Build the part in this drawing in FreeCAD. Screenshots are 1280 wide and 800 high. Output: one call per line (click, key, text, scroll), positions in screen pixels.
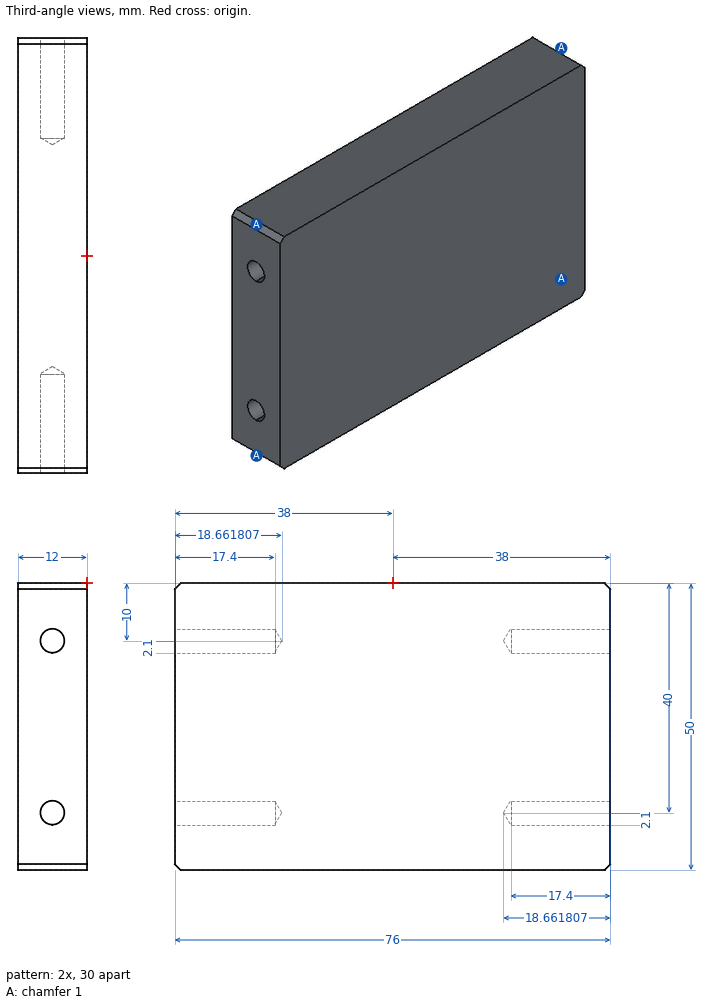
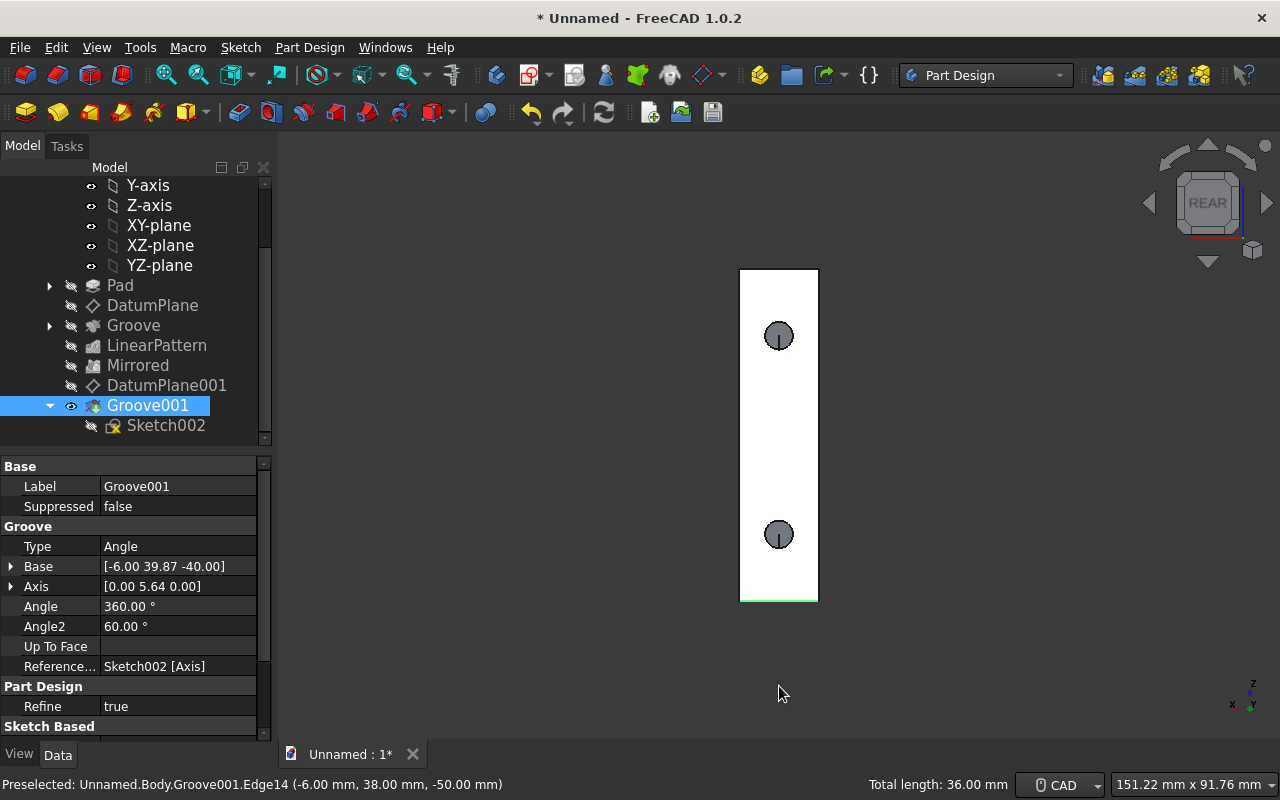
click(779, 268, ctrl)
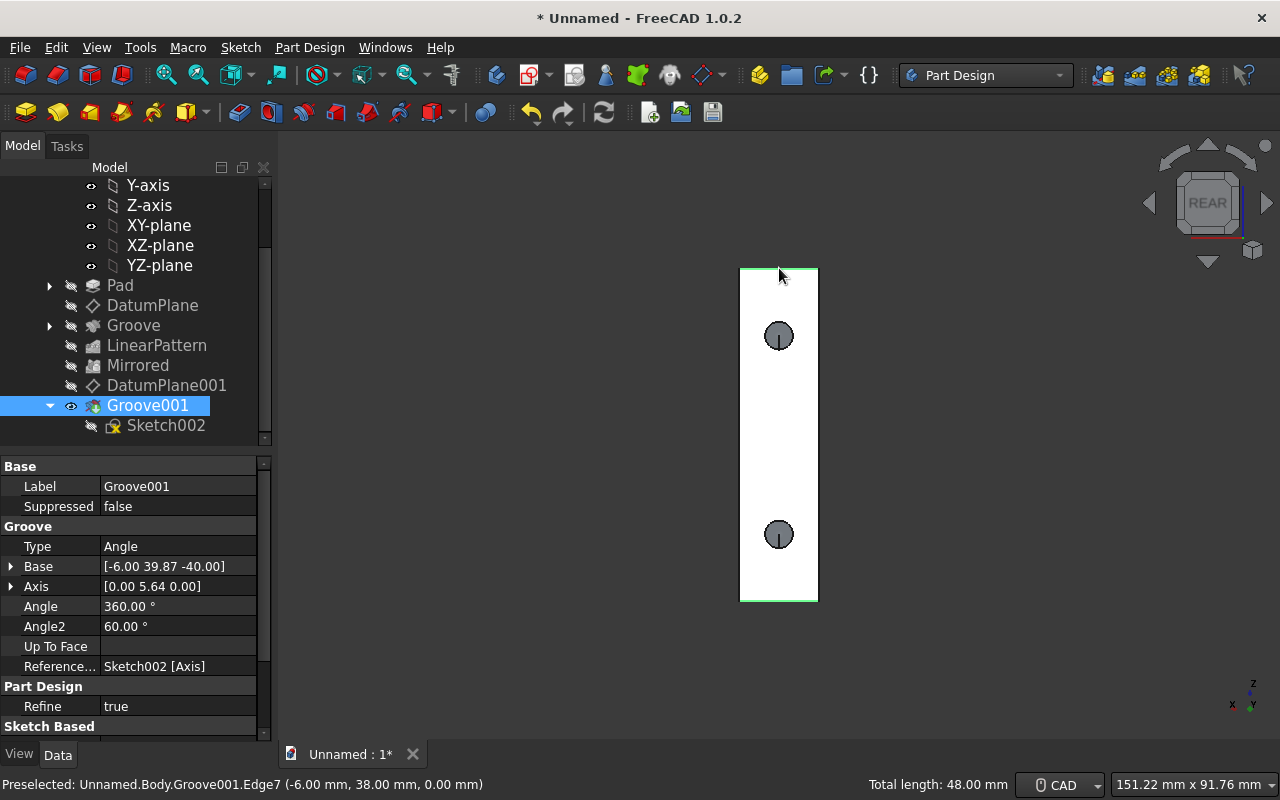
click(58, 76)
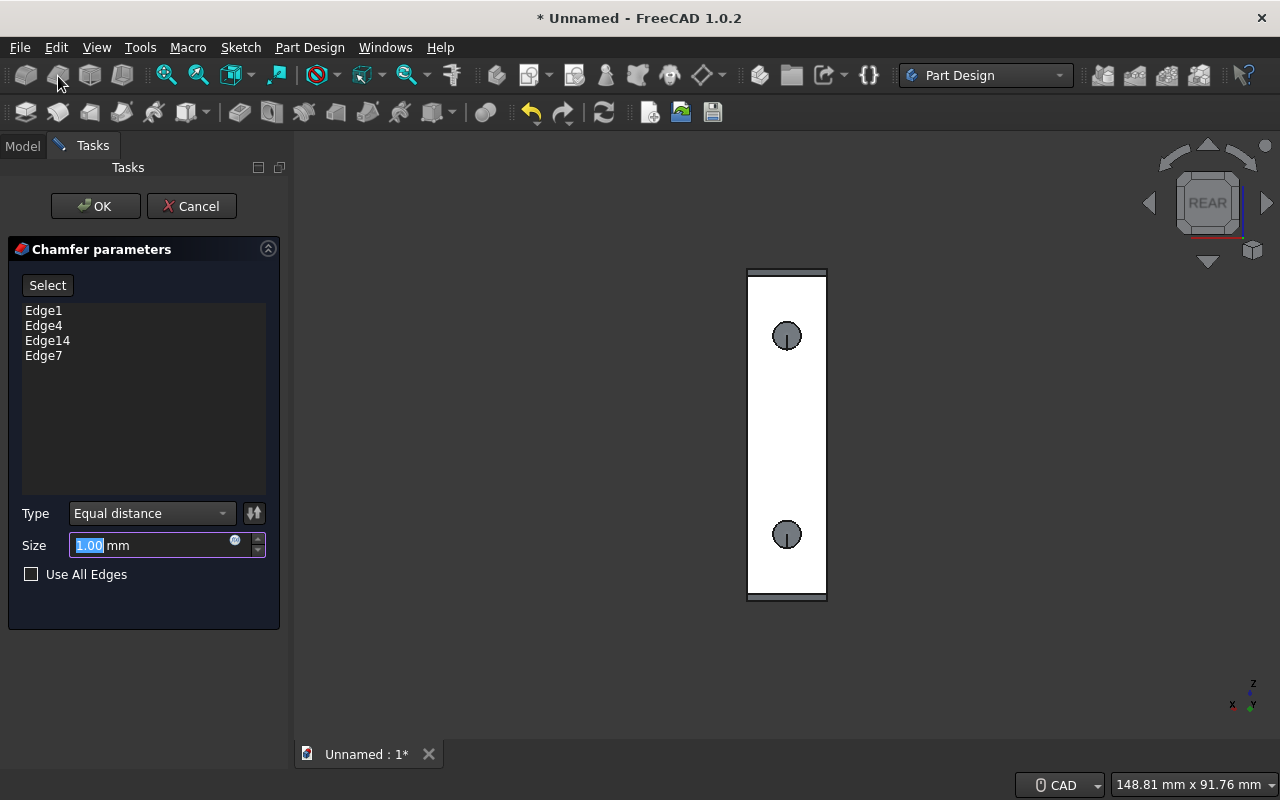
text(1)
key(Tab)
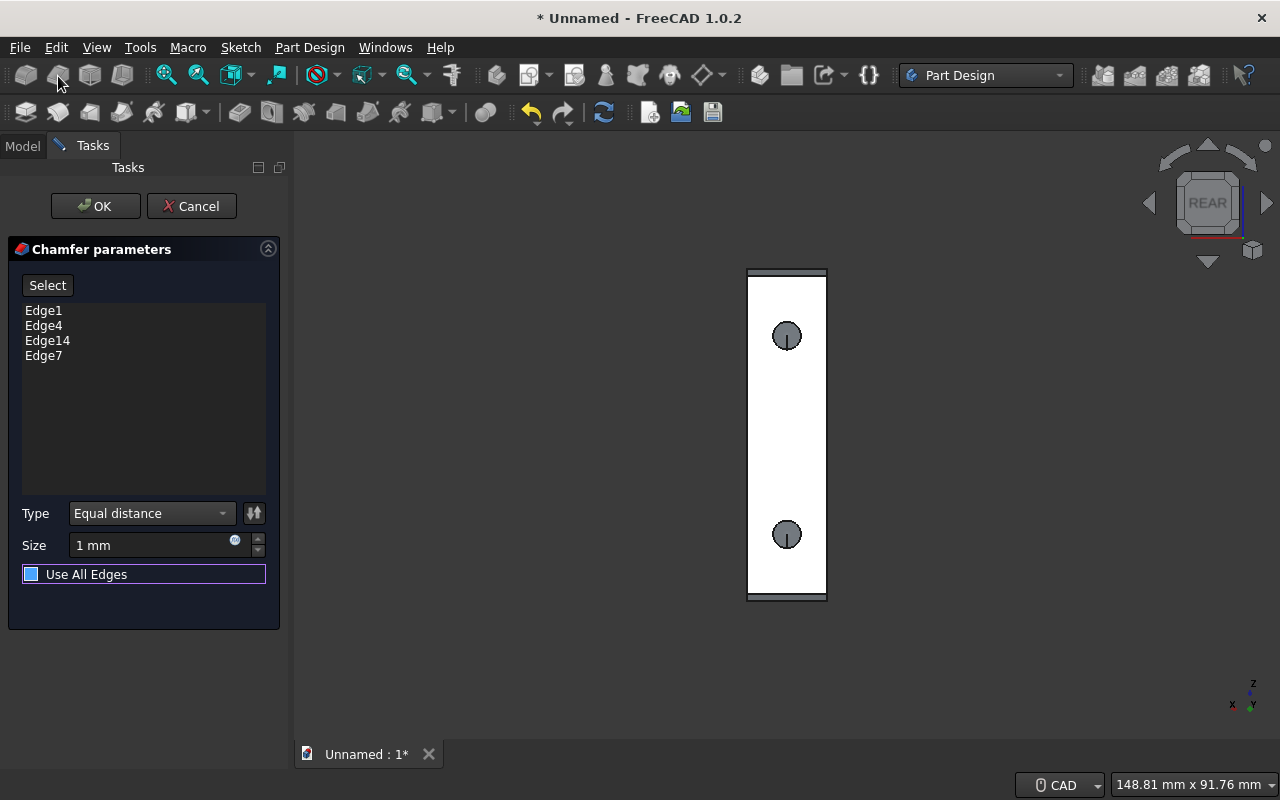
click(96, 206)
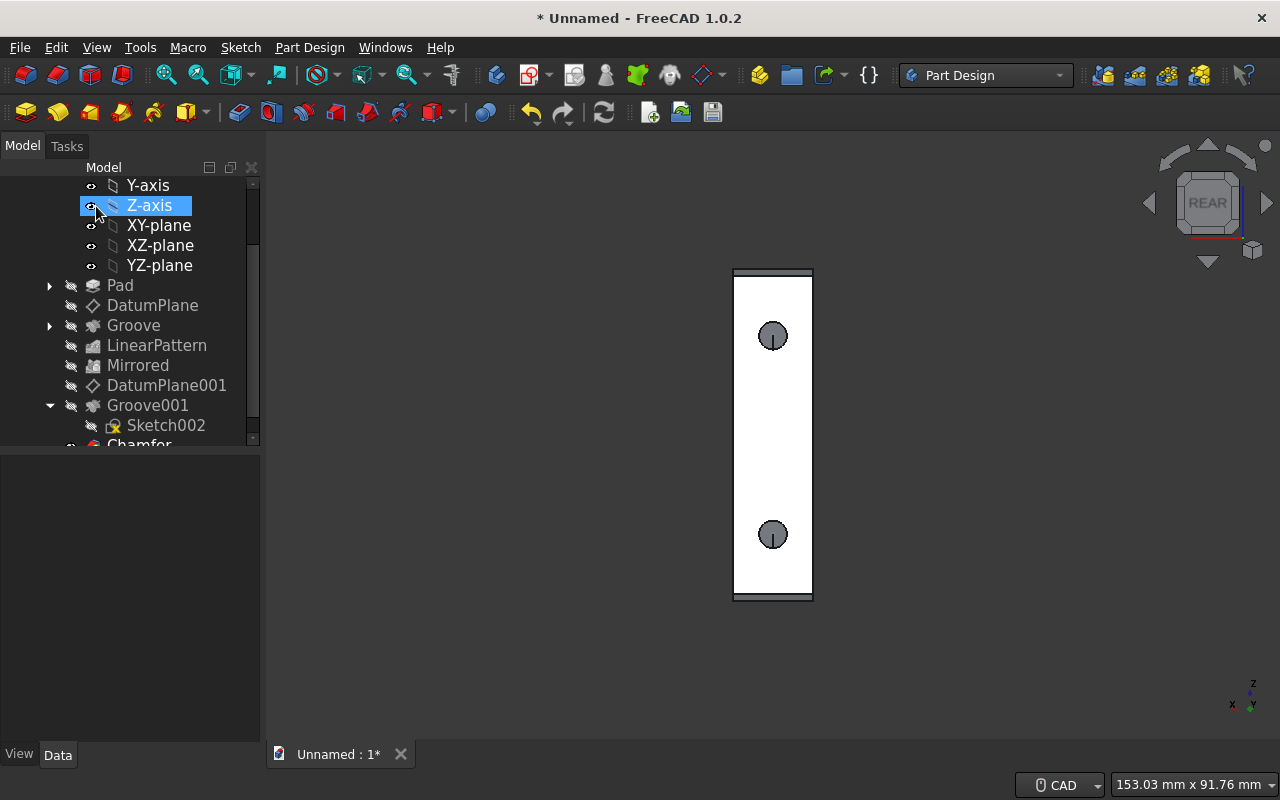
key(0)